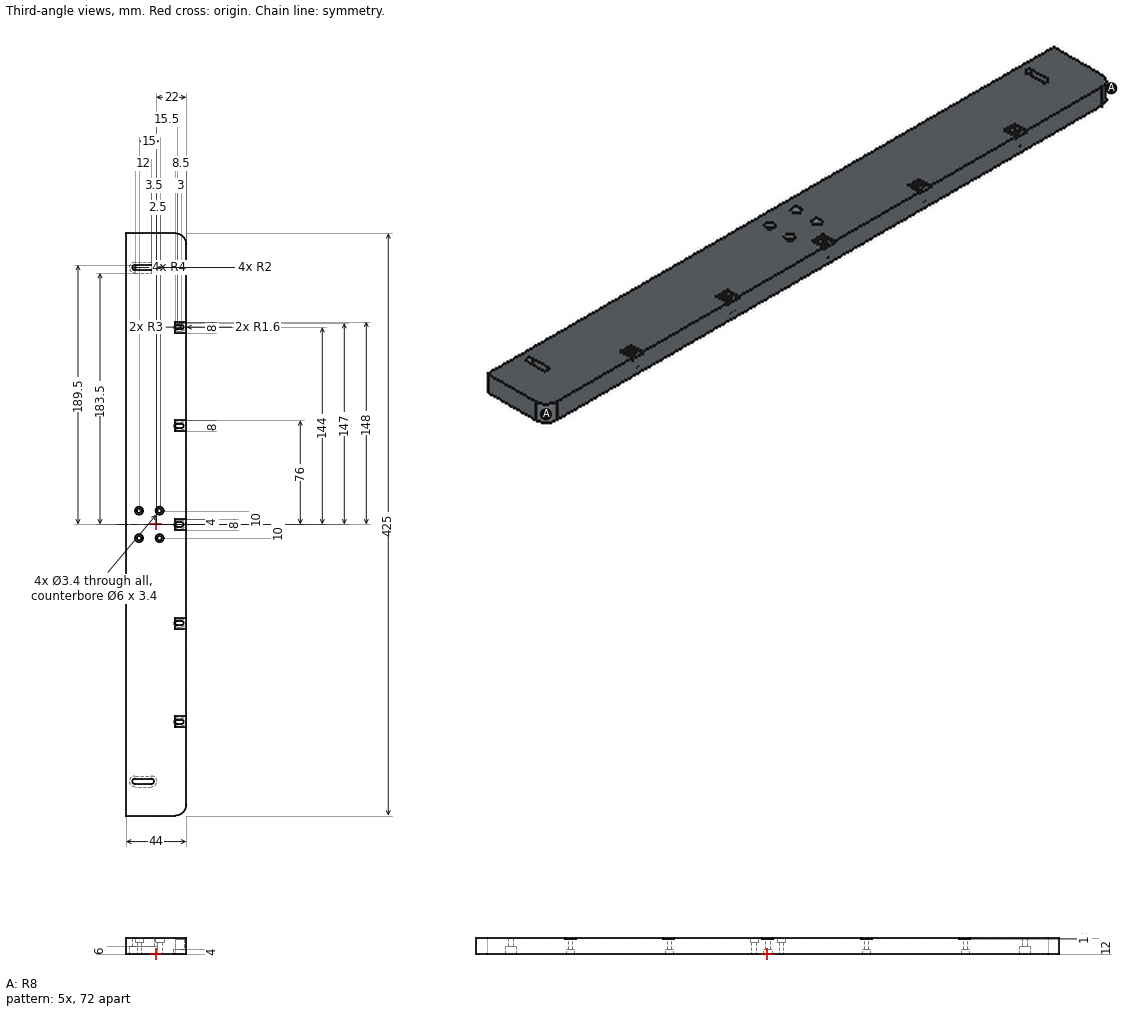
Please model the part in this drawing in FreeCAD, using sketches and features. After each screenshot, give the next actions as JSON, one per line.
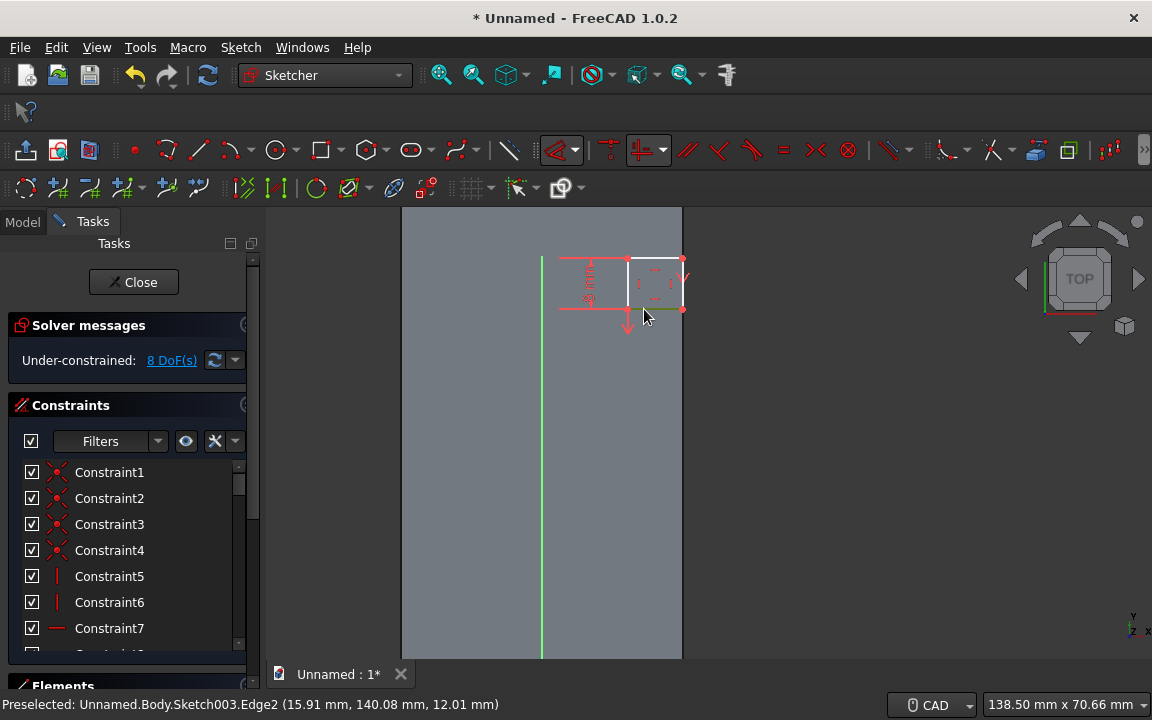
{"action": "left_click", "coordinate": [578, 150]}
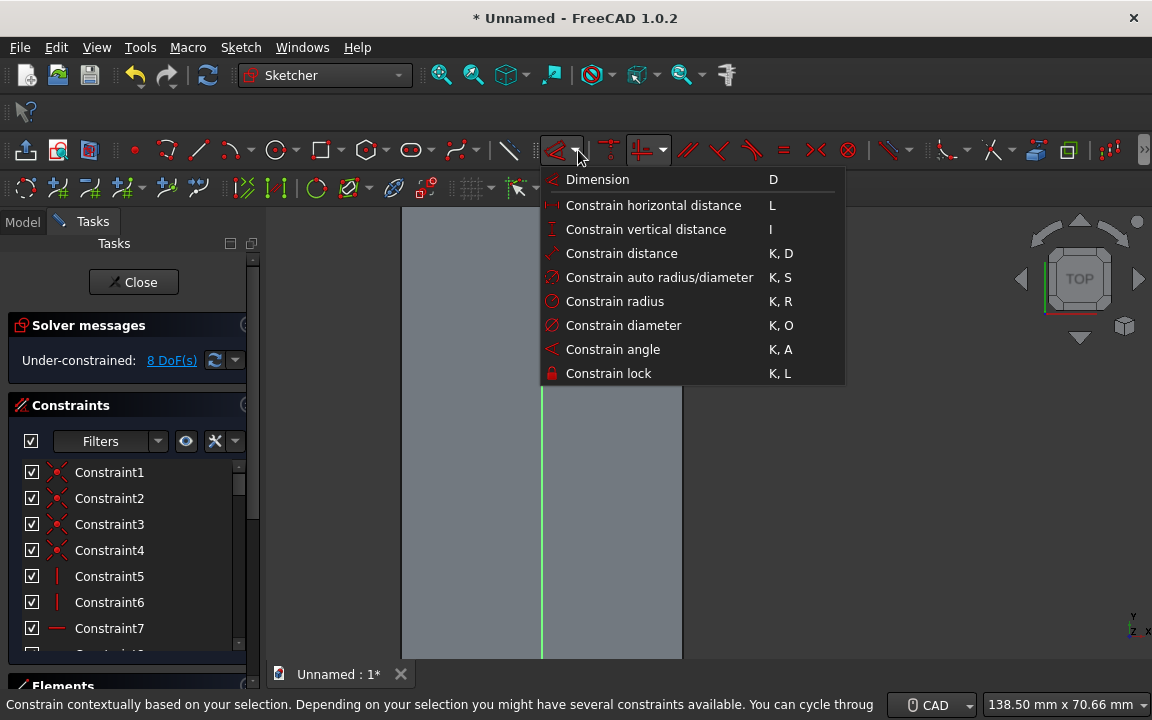
{"action": "left_click", "coordinate": [693, 205]}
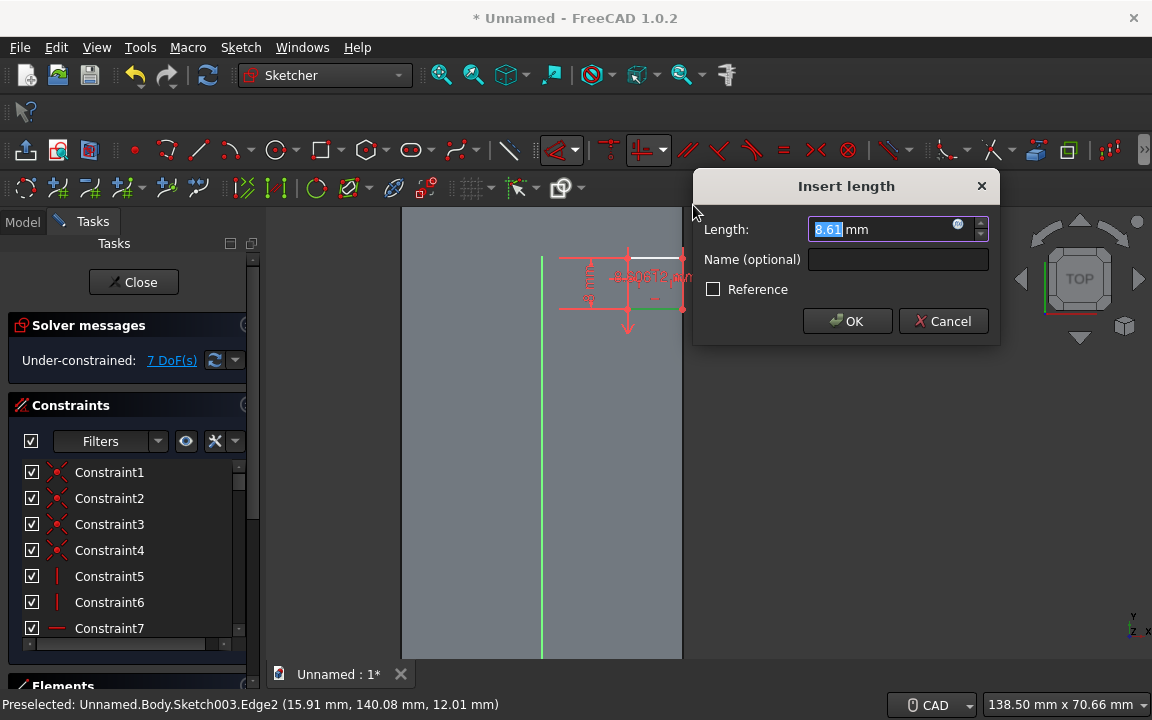
{"action": "type", "text": "8.5"}
{"action": "key", "text": "Return"}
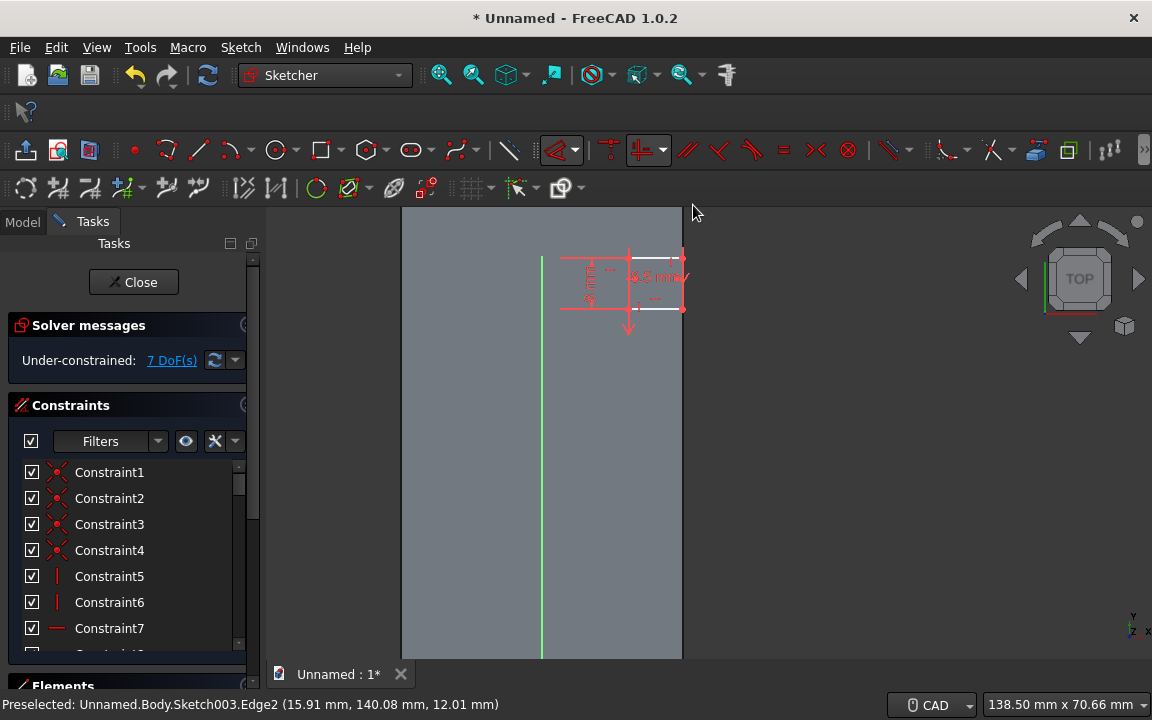
{"action": "scroll", "coordinate": [645, 312], "scroll_direction": "down", "scroll_amount": 10}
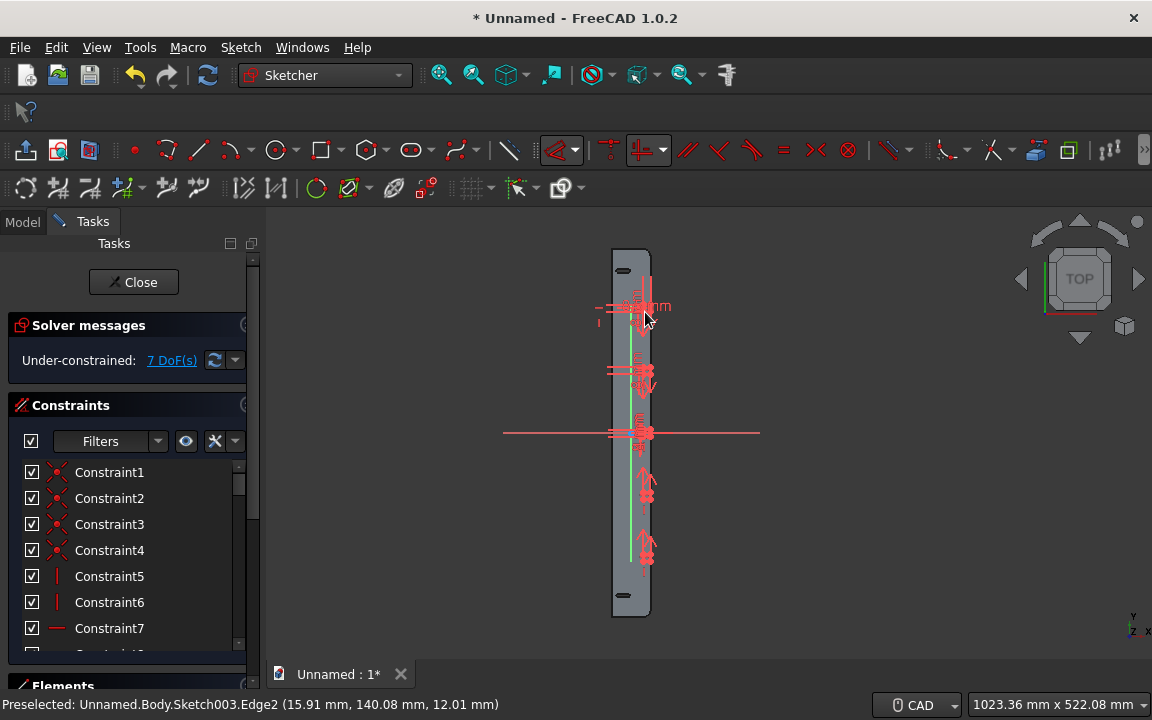
{"action": "scroll", "coordinate": [645, 374], "scroll_direction": "up", "scroll_amount": 10}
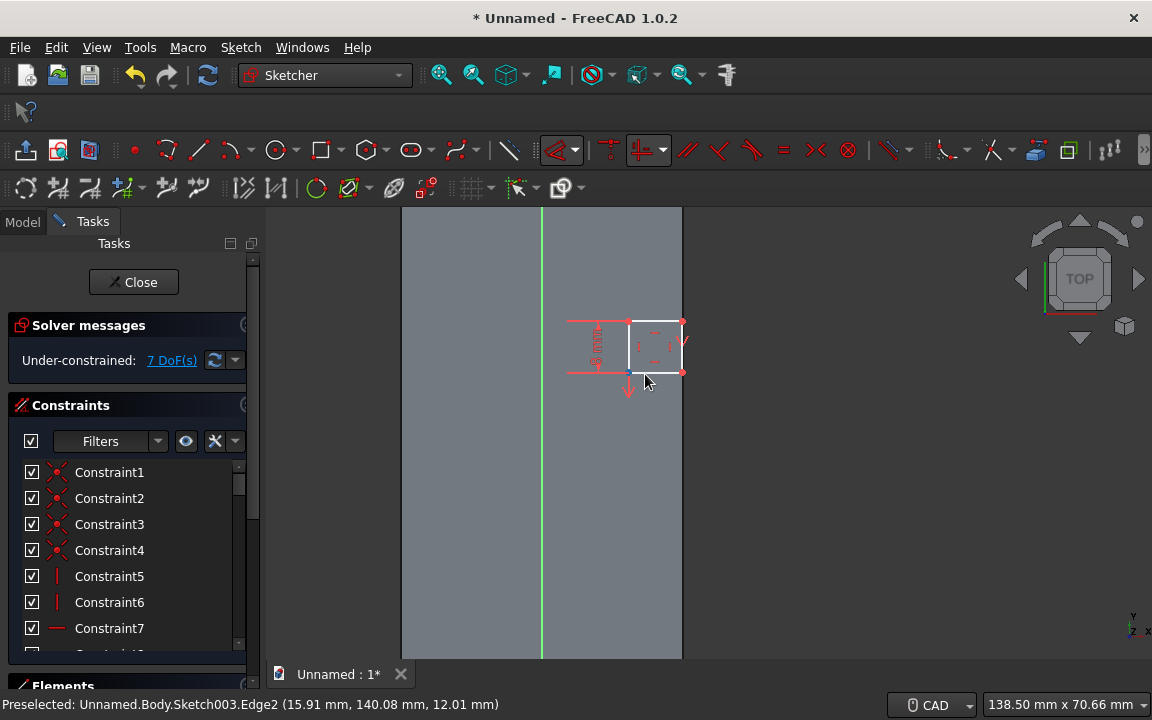
{"action": "left_click", "coordinate": [645, 373]}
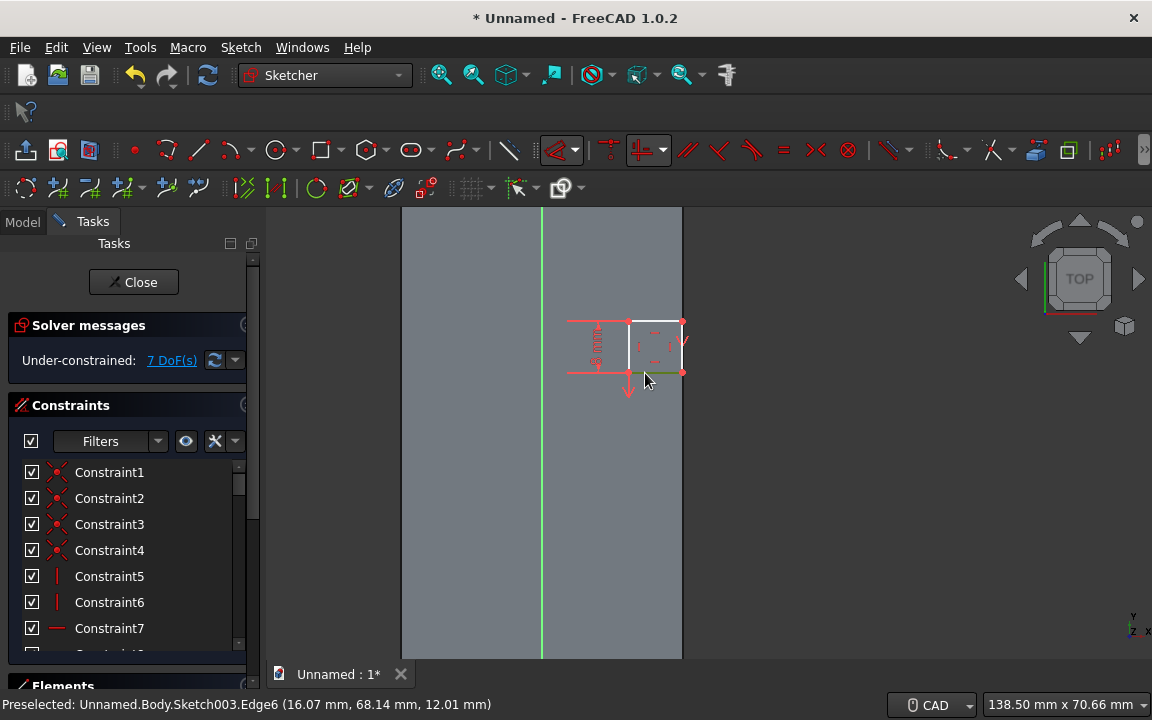
{"action": "key", "text": "l"}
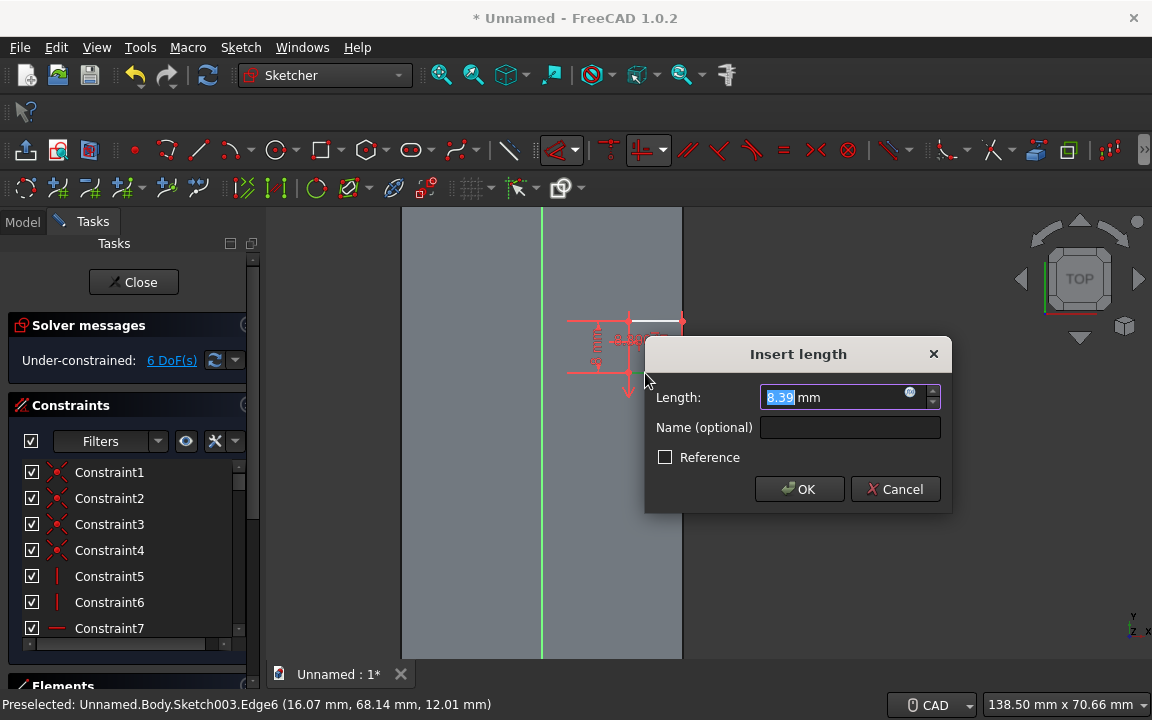
{"action": "type", "text": "8.5"}
{"action": "key", "text": "Return"}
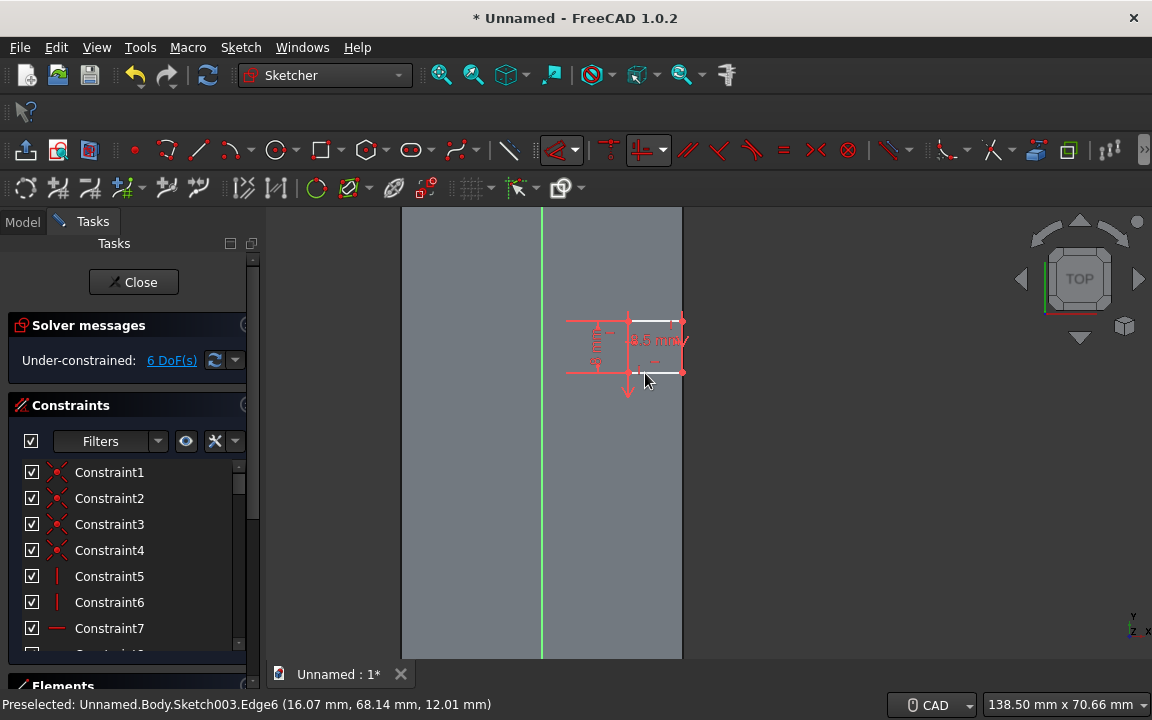
{"action": "scroll", "coordinate": [645, 374], "scroll_direction": "down", "scroll_amount": 10}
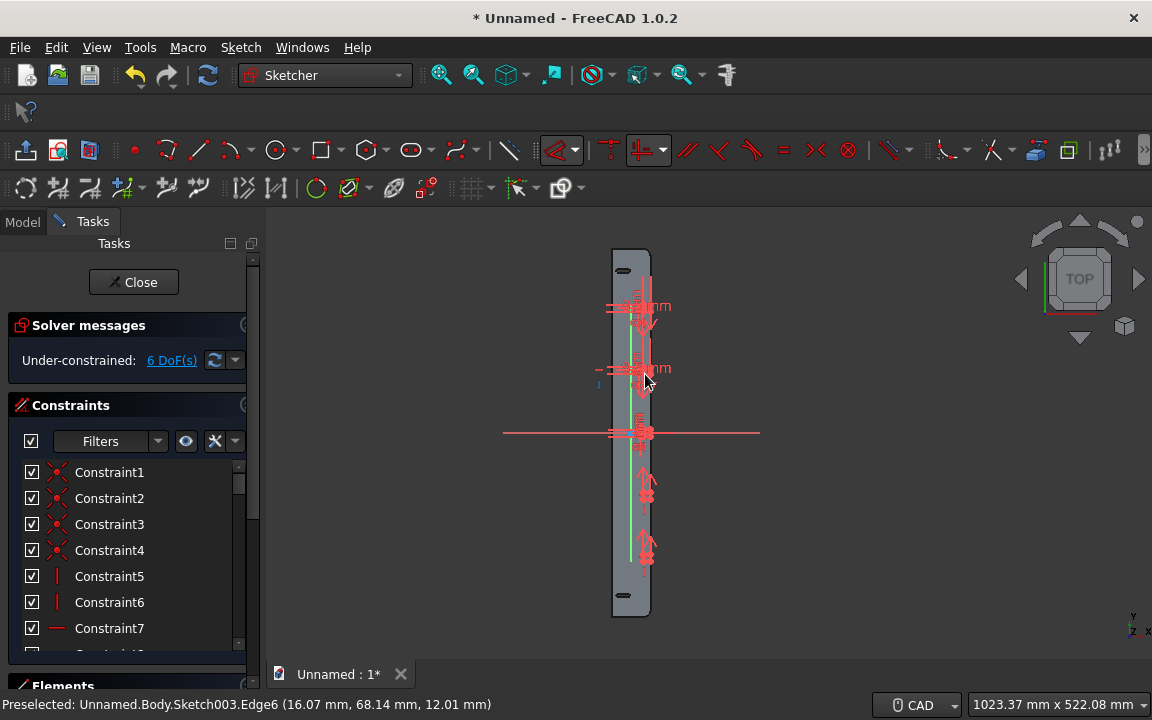
{"action": "scroll", "coordinate": [645, 437], "scroll_direction": "up", "scroll_amount": 10}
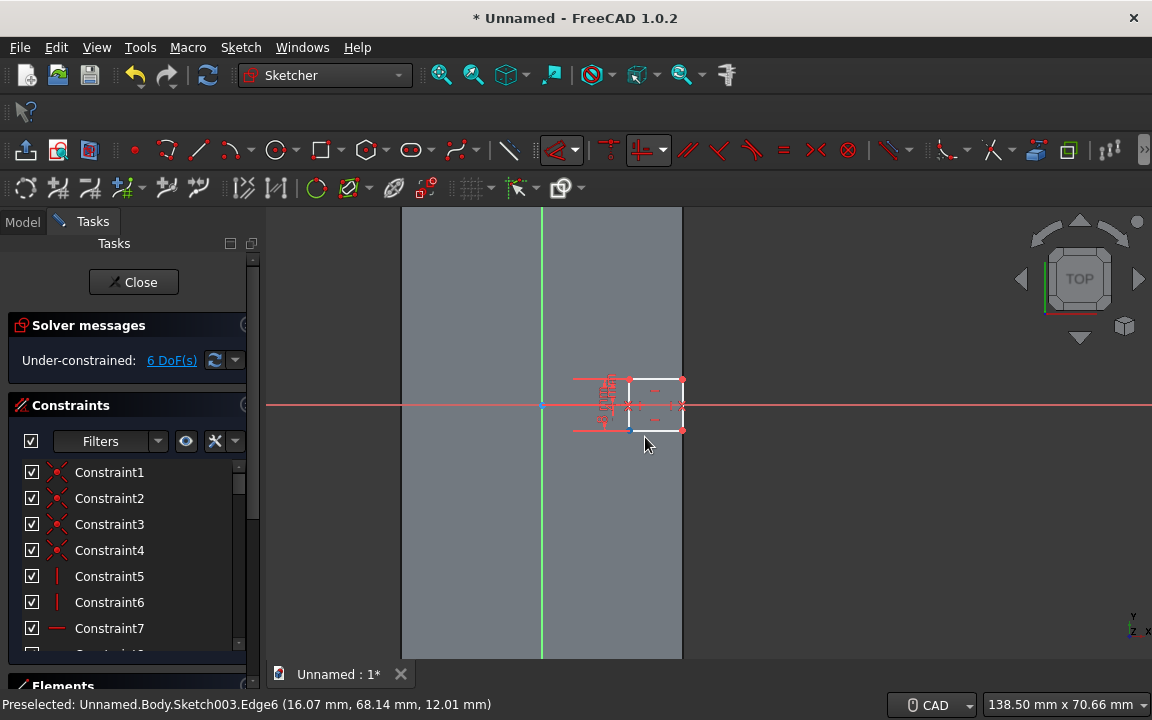
{"action": "left_click", "coordinate": [645, 431]}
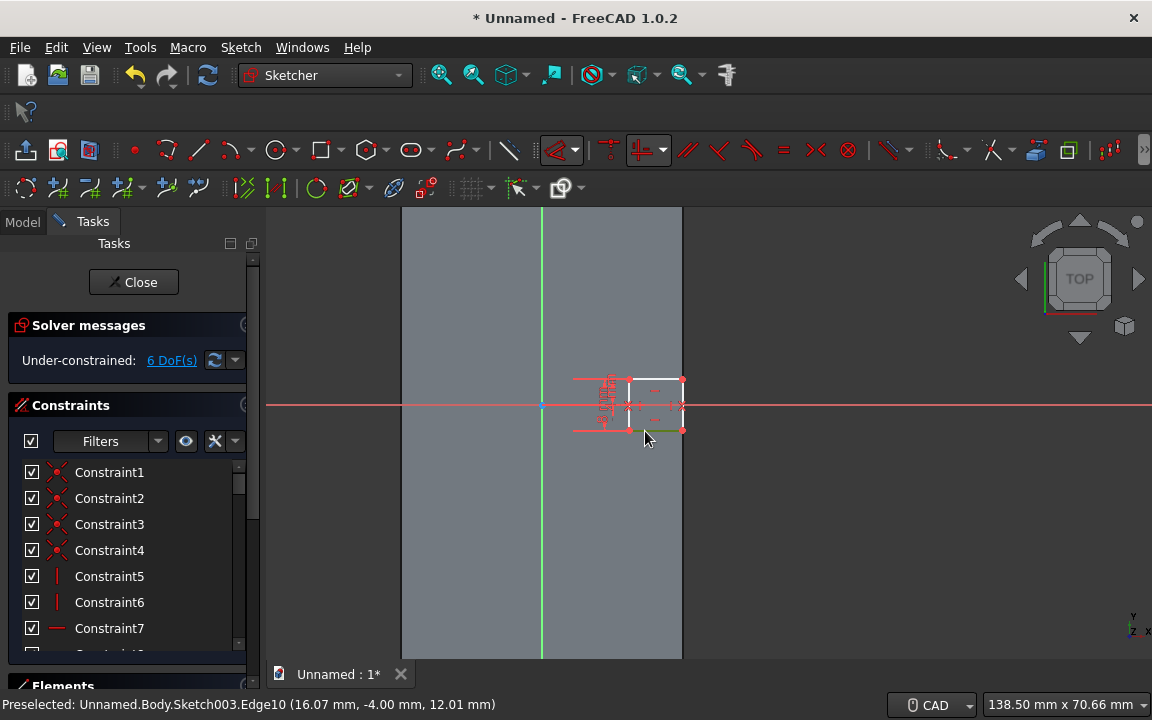
{"action": "key", "text": "l"}